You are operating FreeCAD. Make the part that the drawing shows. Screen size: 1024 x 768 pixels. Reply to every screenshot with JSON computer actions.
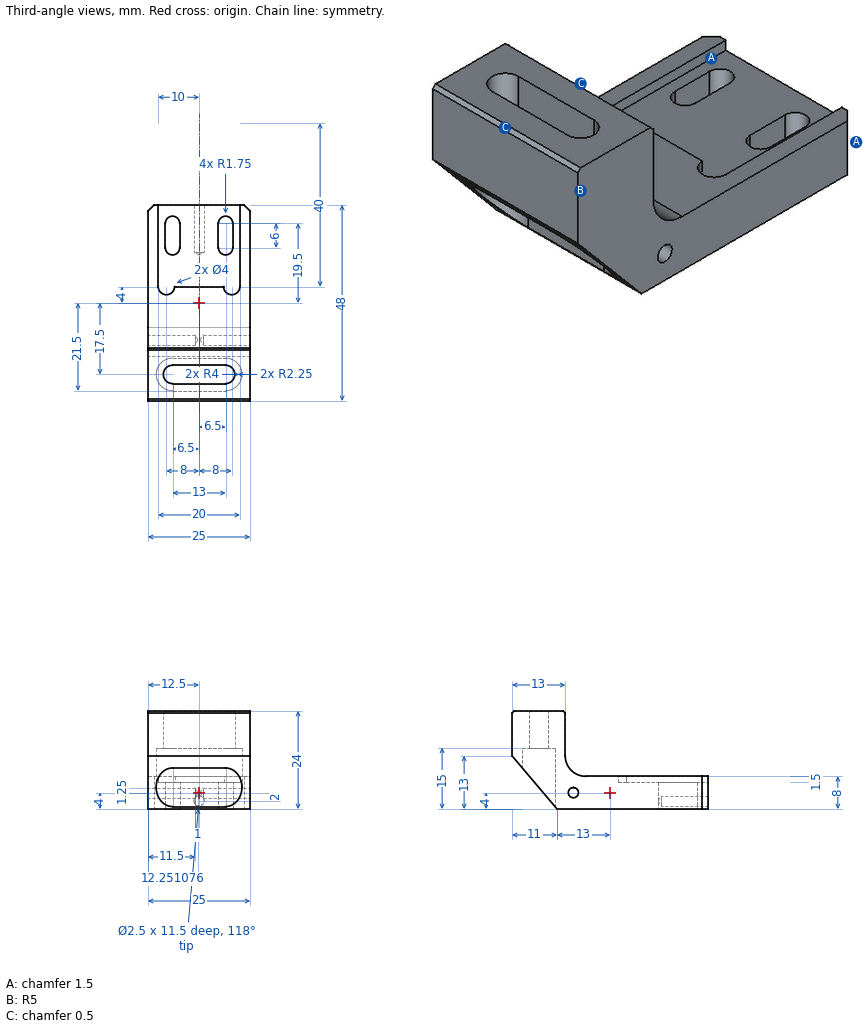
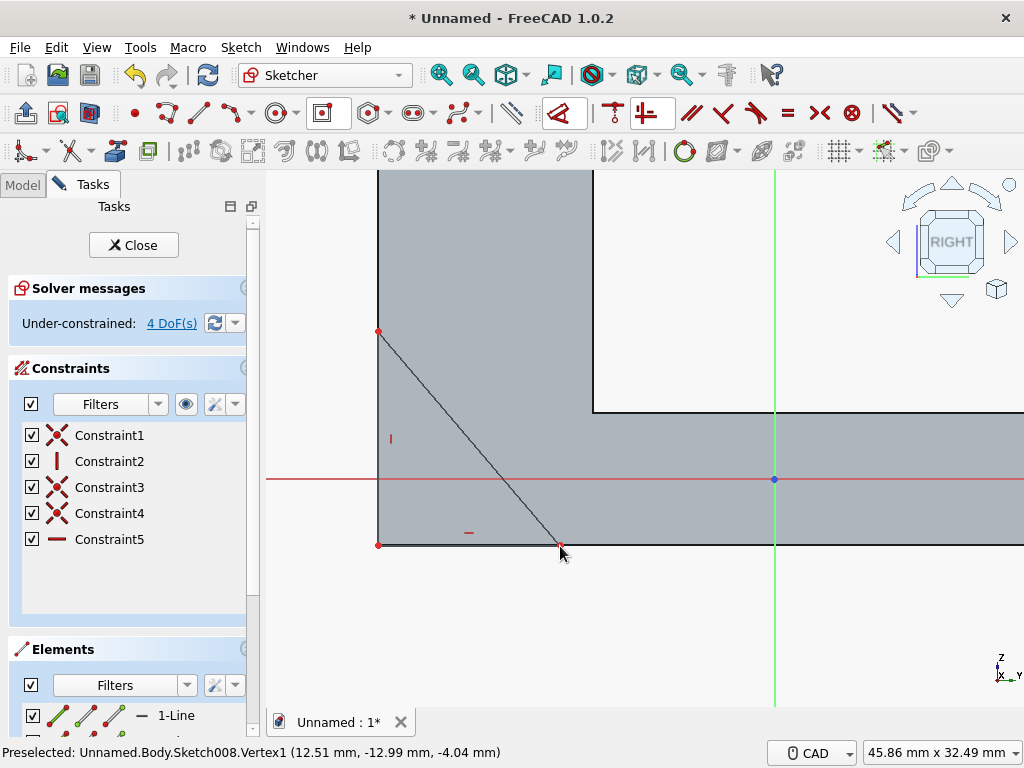
{"action": "left_click", "coordinate": [378, 396]}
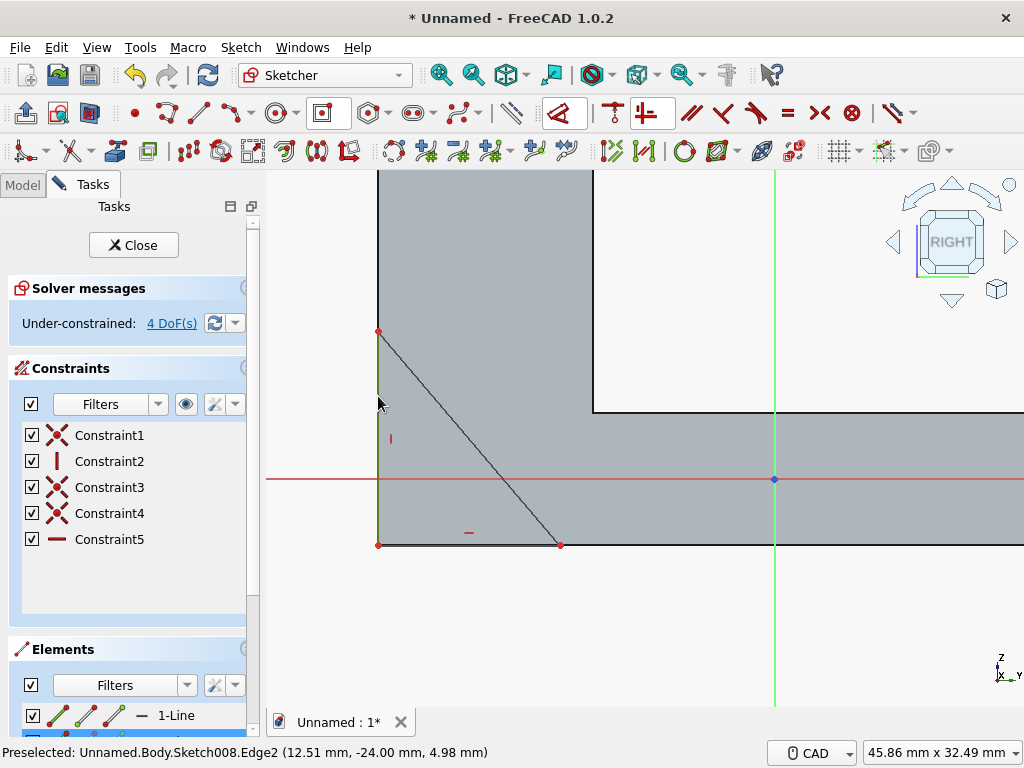
{"action": "key", "text": "i"}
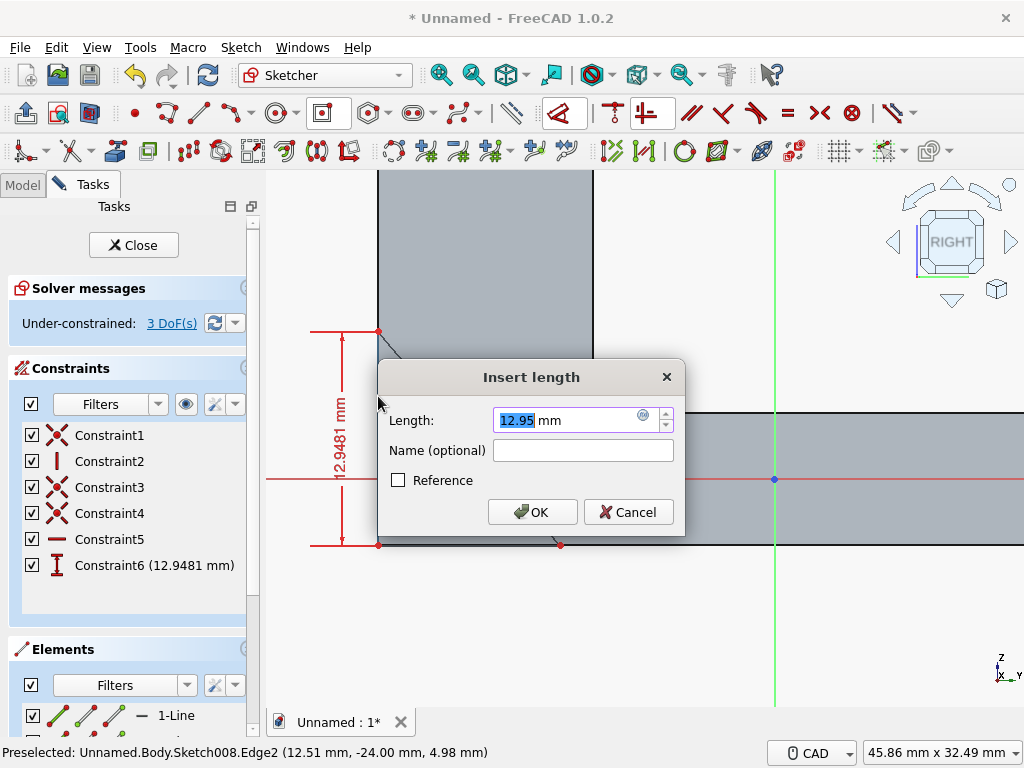
{"action": "type", "text": "13"}
{"action": "key", "text": "Return"}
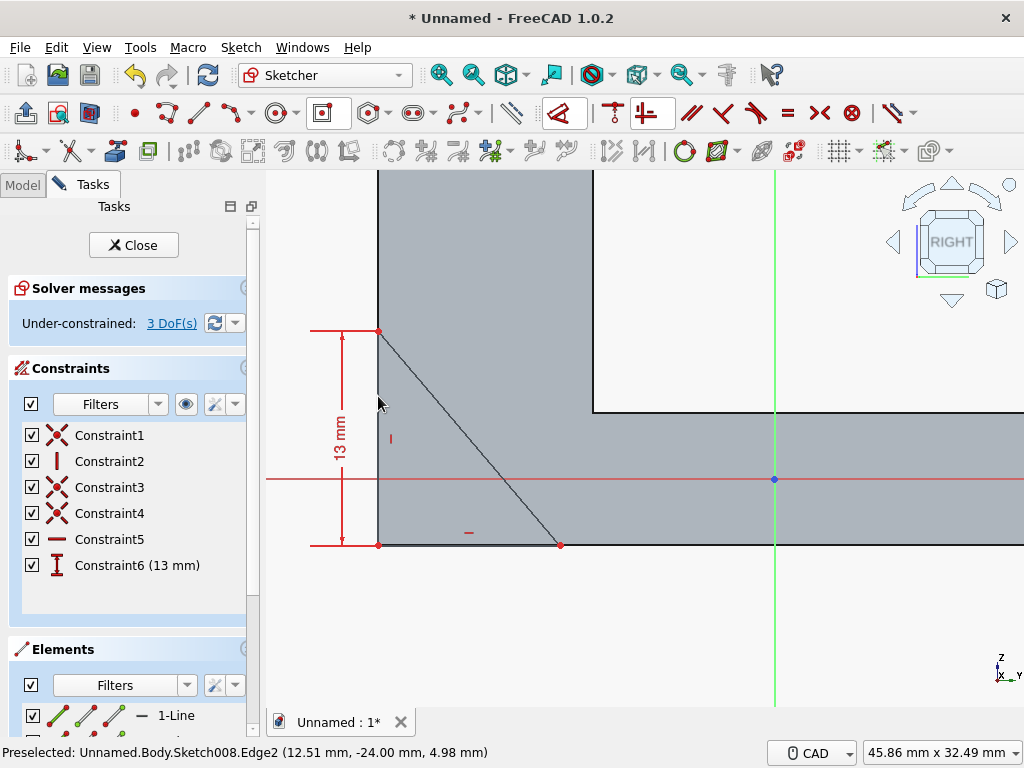
{"action": "left_click", "coordinate": [433, 546]}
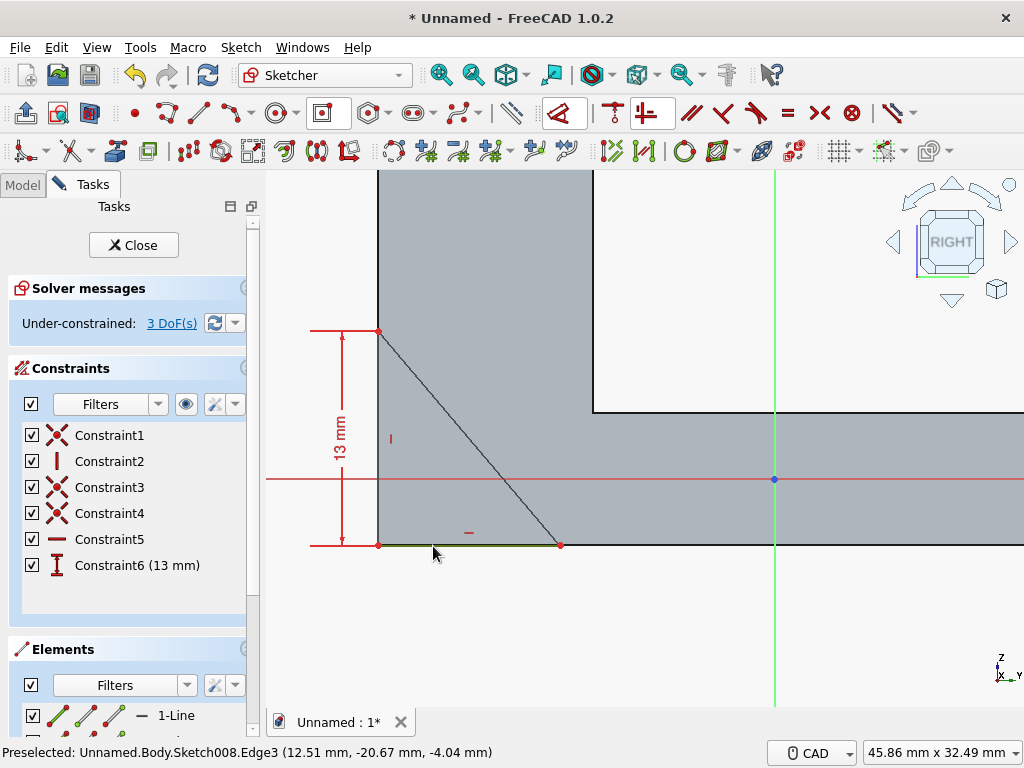
{"action": "key", "text": "l"}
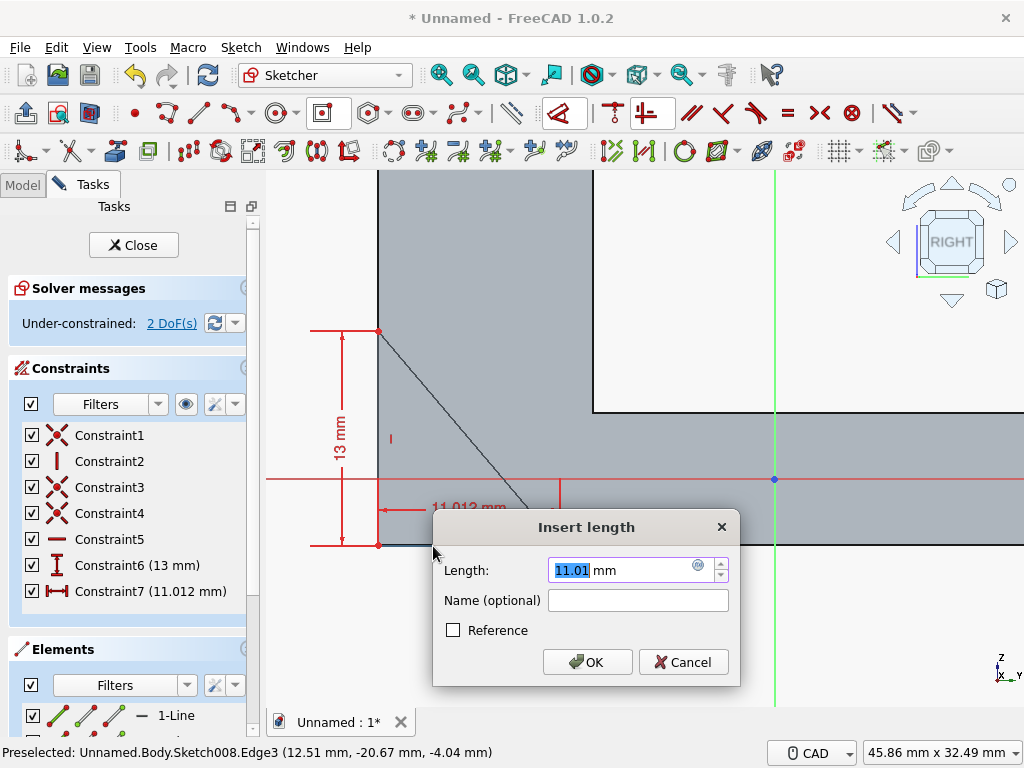
{"action": "type", "text": "11"}
{"action": "key", "text": "Return"}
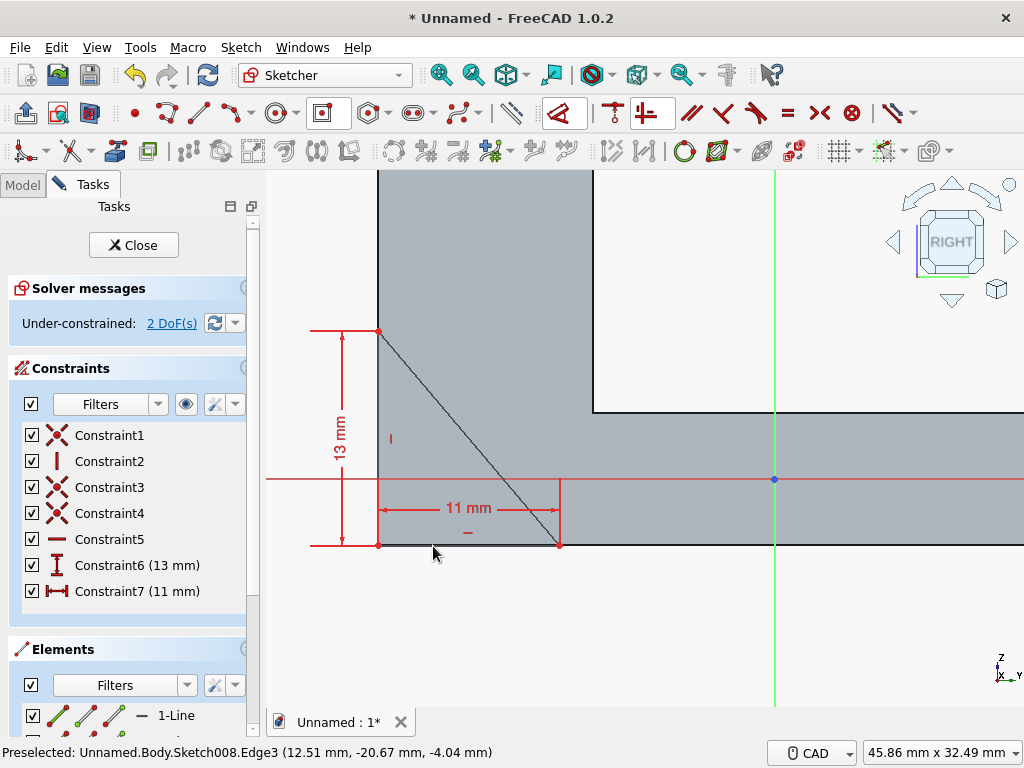
{"action": "left_click", "coordinate": [560, 546]}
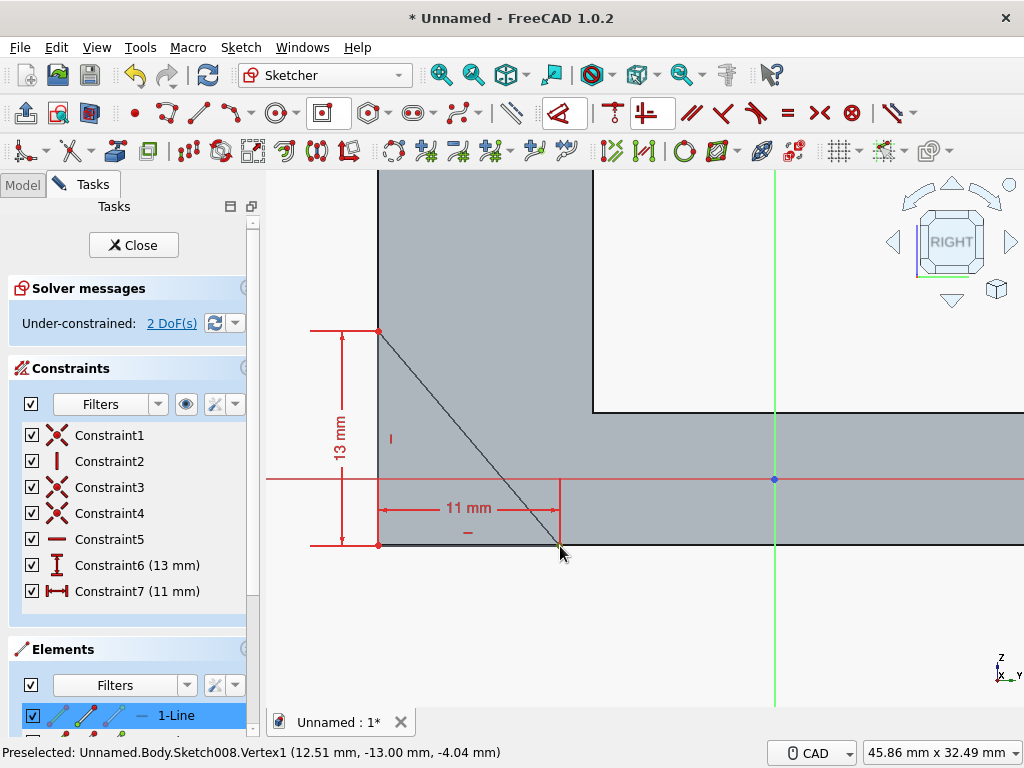
{"action": "left_click", "coordinate": [582, 114]}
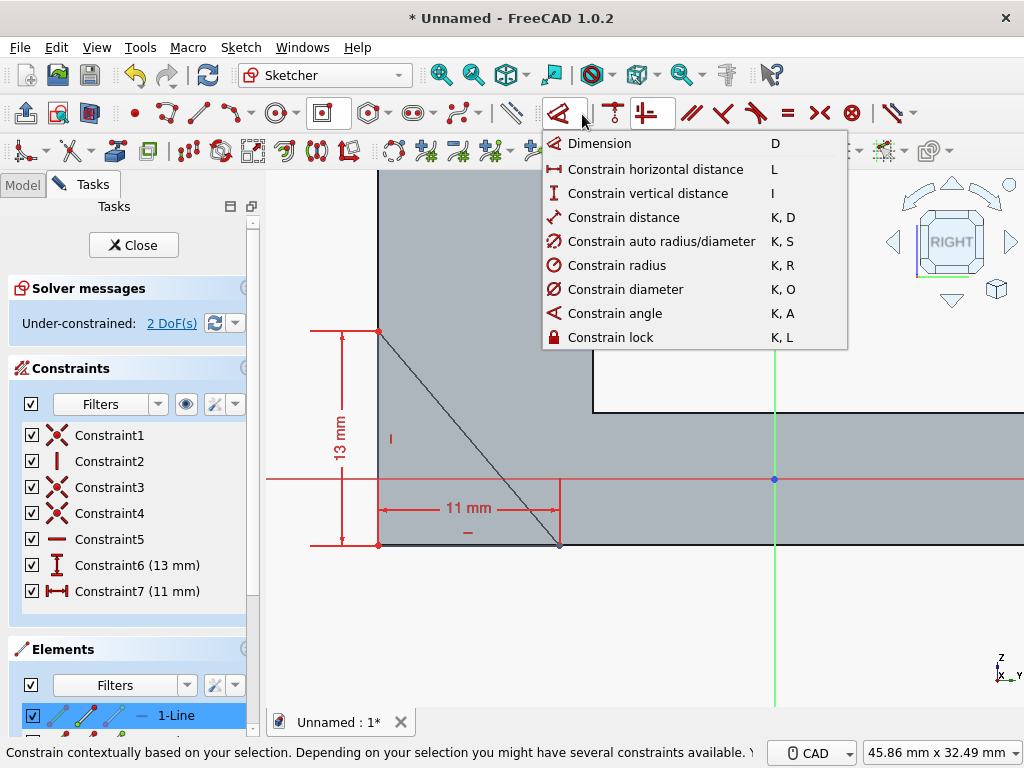
{"action": "left_click", "coordinate": [695, 193]}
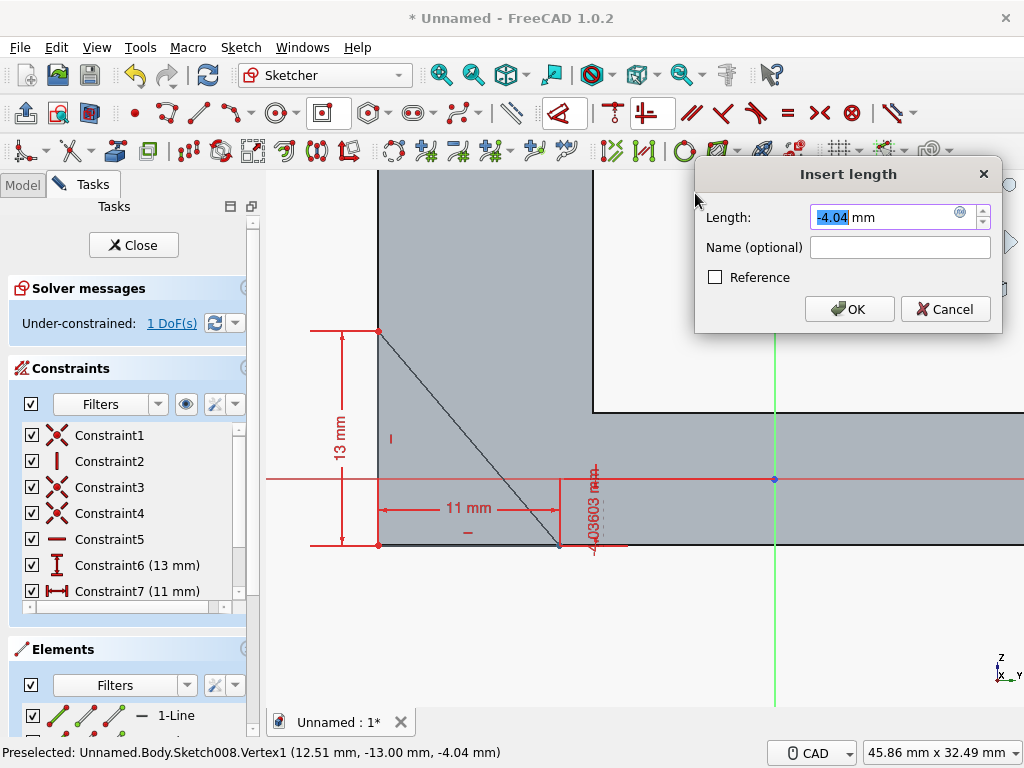
{"action": "type", "text": "-4"}
{"action": "key", "text": "Return"}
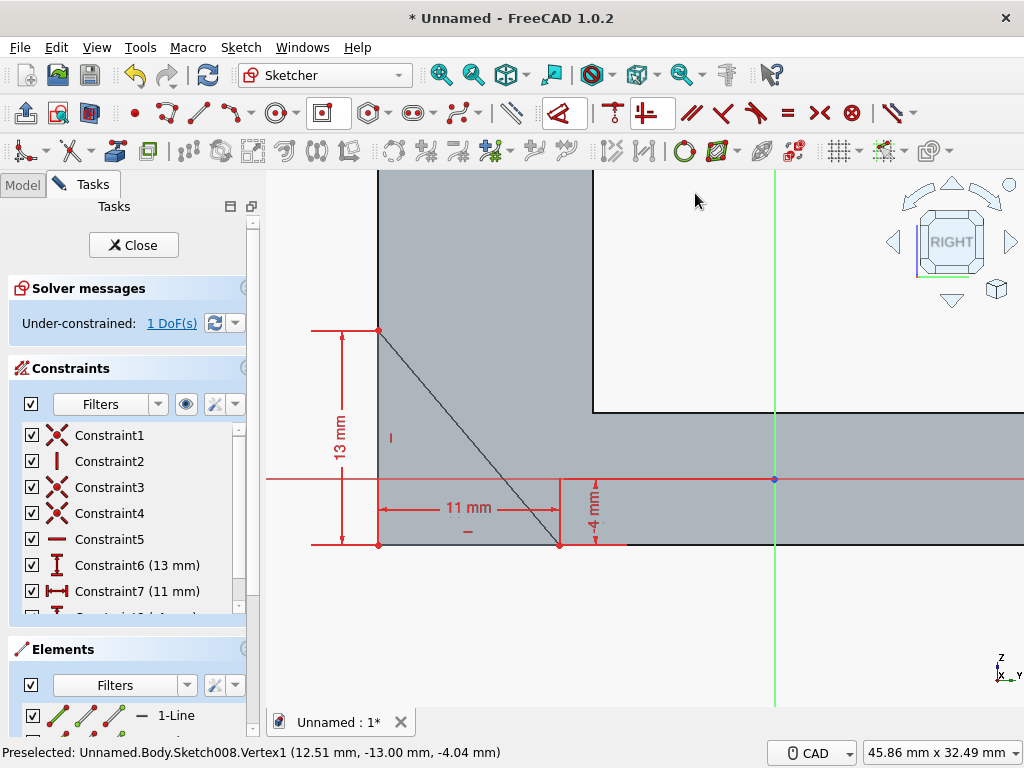
{"action": "left_click", "coordinate": [560, 545]}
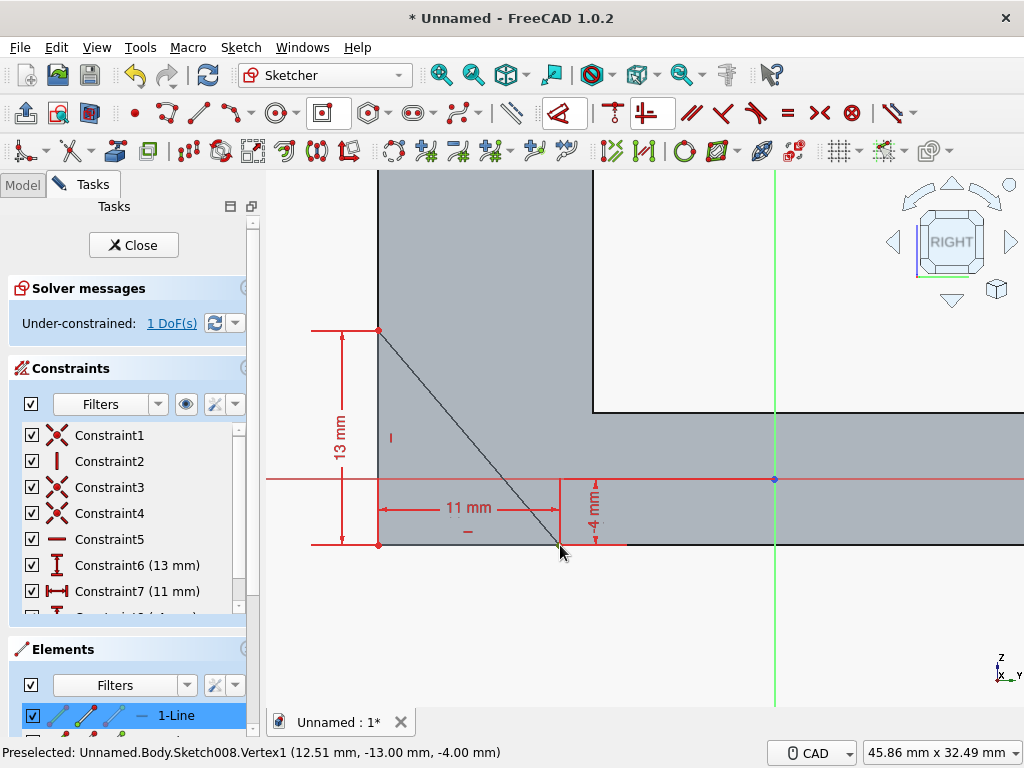
{"action": "left_click", "coordinate": [582, 114]}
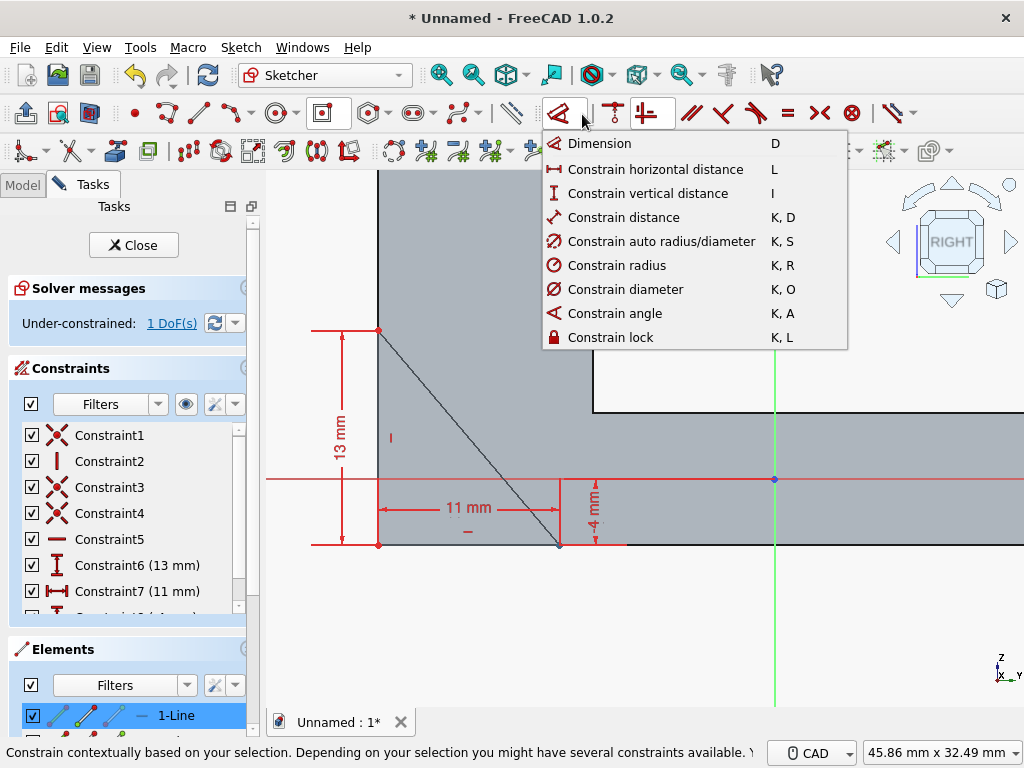
{"action": "left_click", "coordinate": [695, 169]}